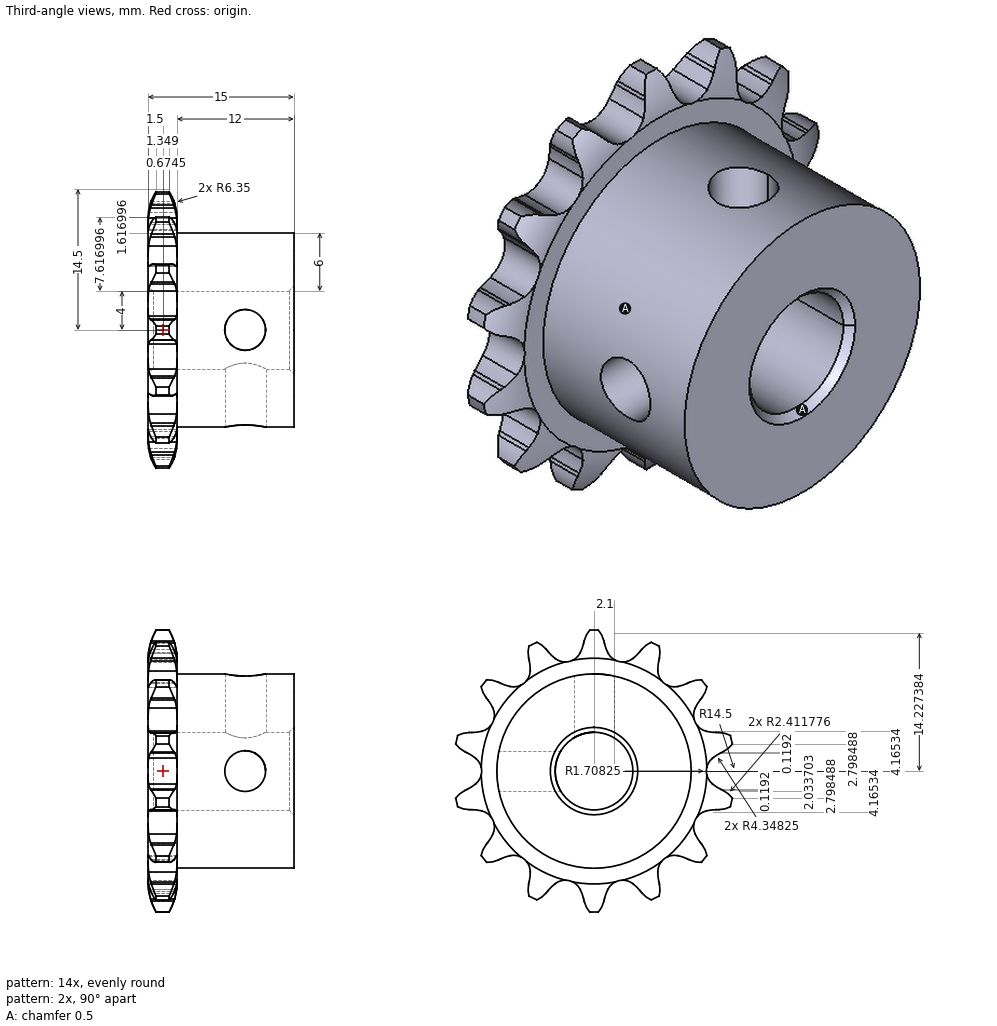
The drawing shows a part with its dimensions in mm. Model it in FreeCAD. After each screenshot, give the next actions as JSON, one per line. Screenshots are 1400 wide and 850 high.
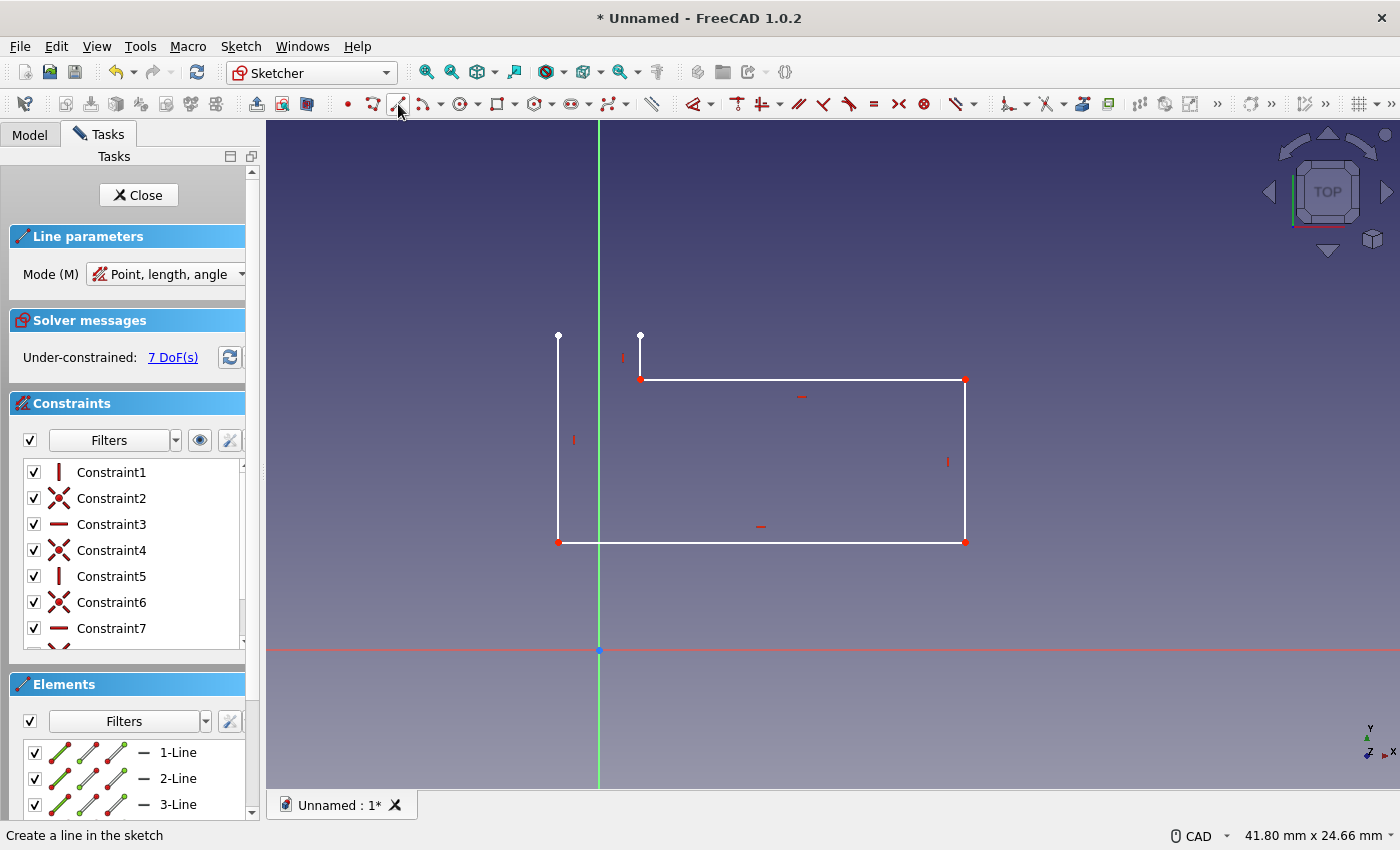
{"action": "left_click", "coordinate": [617, 257]}
{"action": "left_click", "coordinate": [581, 257]}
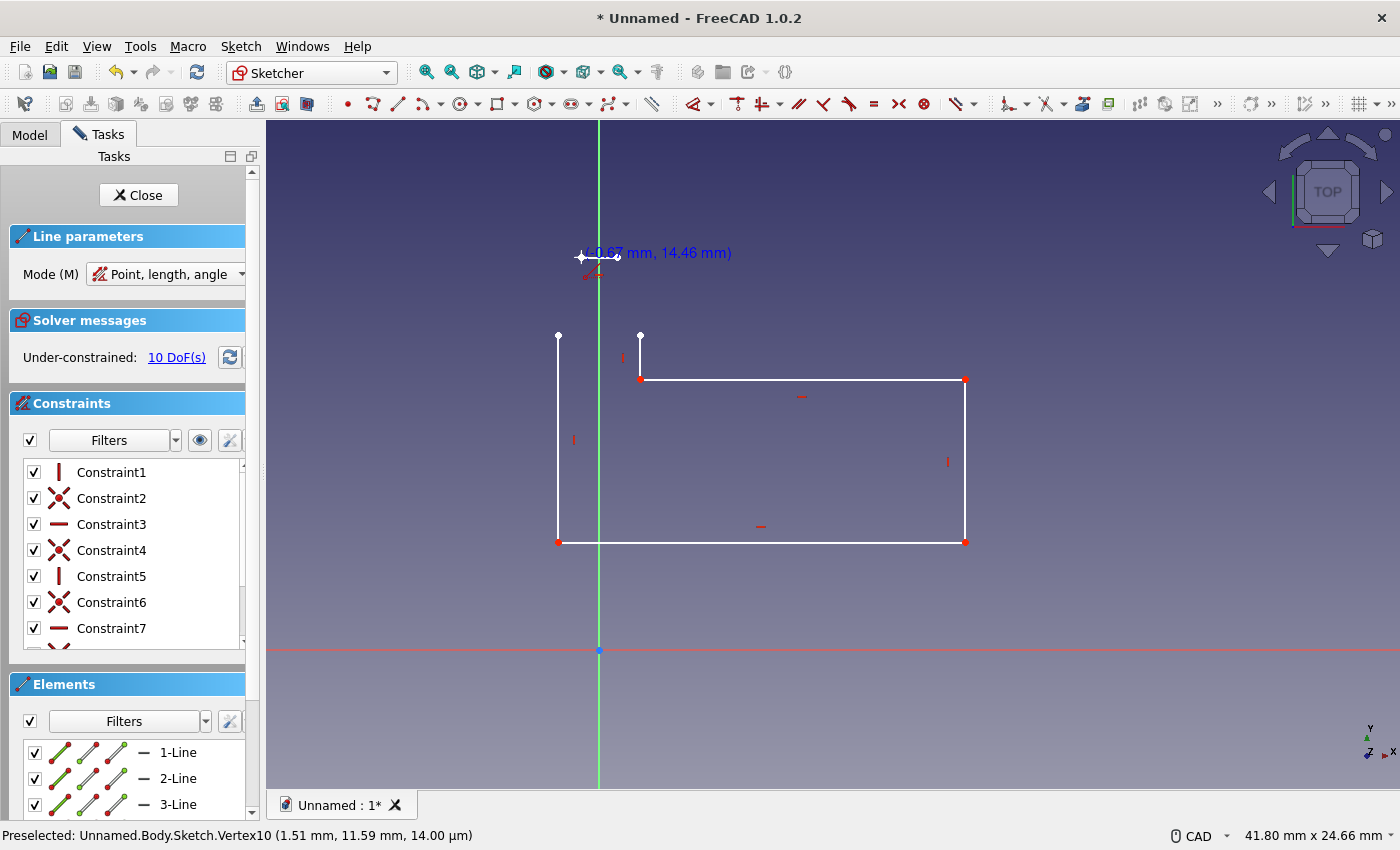
{"action": "key", "text": "g 3 a"}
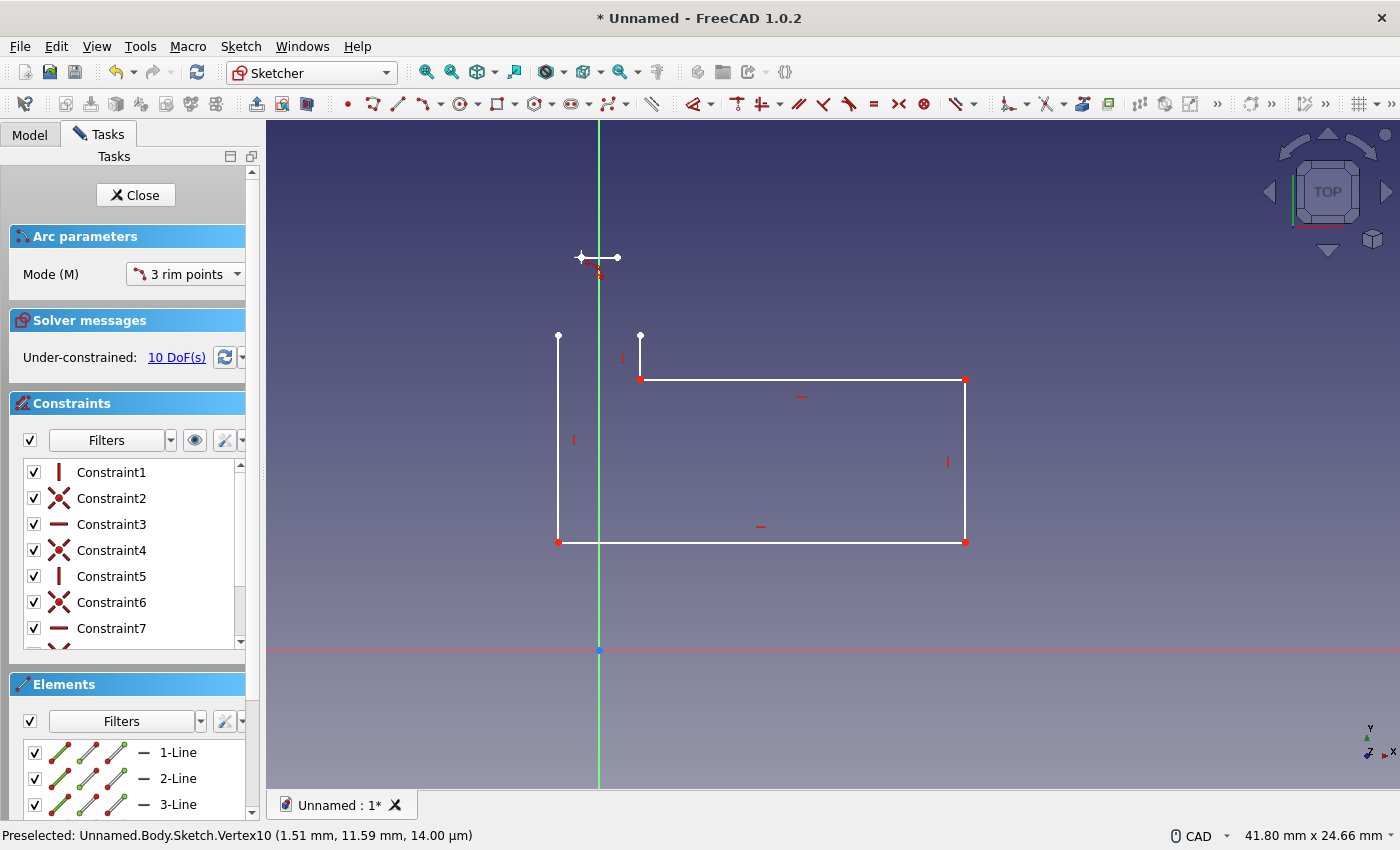
{"action": "left_click", "coordinate": [640, 336]}
{"action": "left_click", "coordinate": [617, 258]}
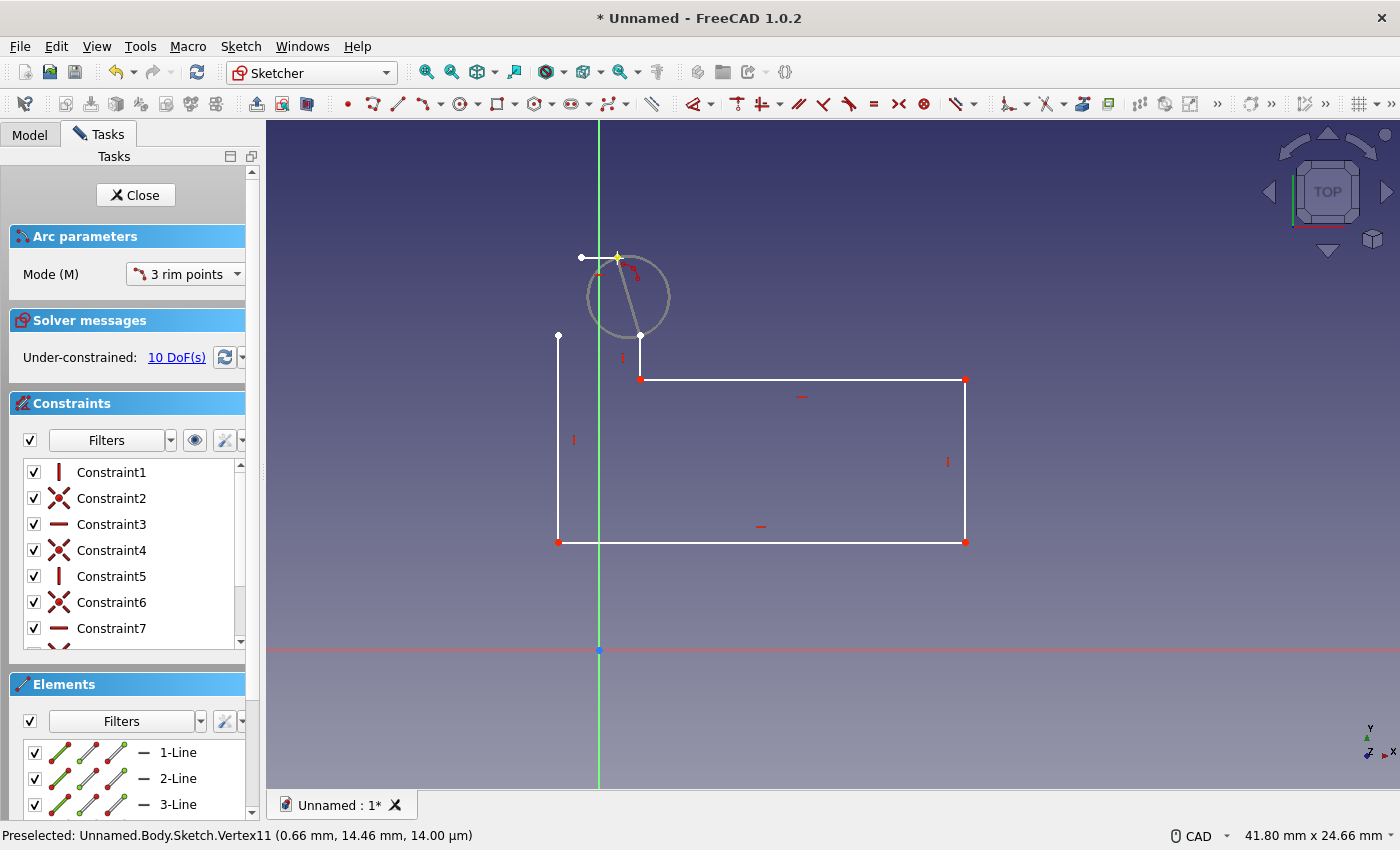
{"action": "scroll", "coordinate": [633, 295], "scroll_direction": "up", "scroll_amount": 6}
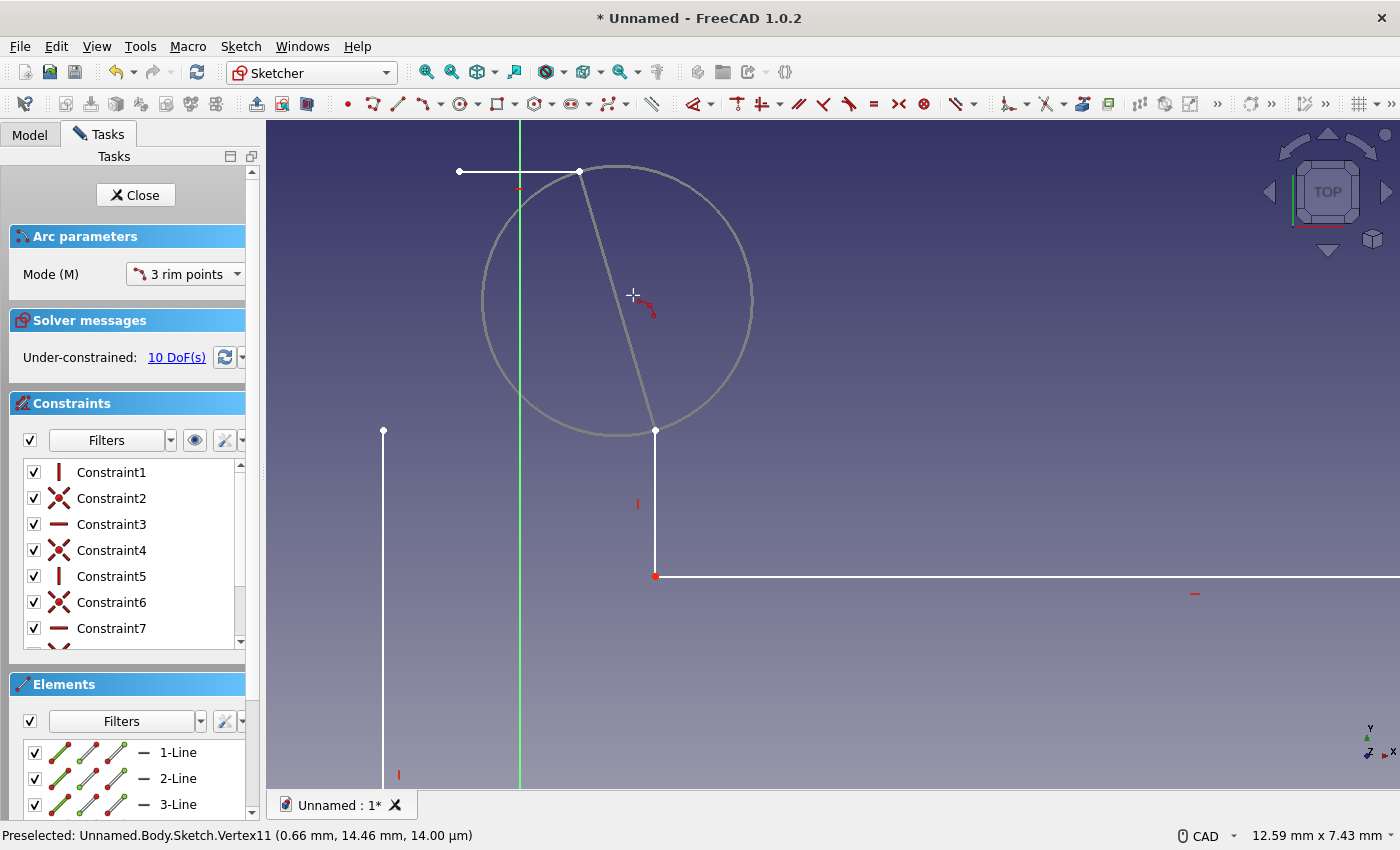
{"action": "left_click", "coordinate": [633, 293]}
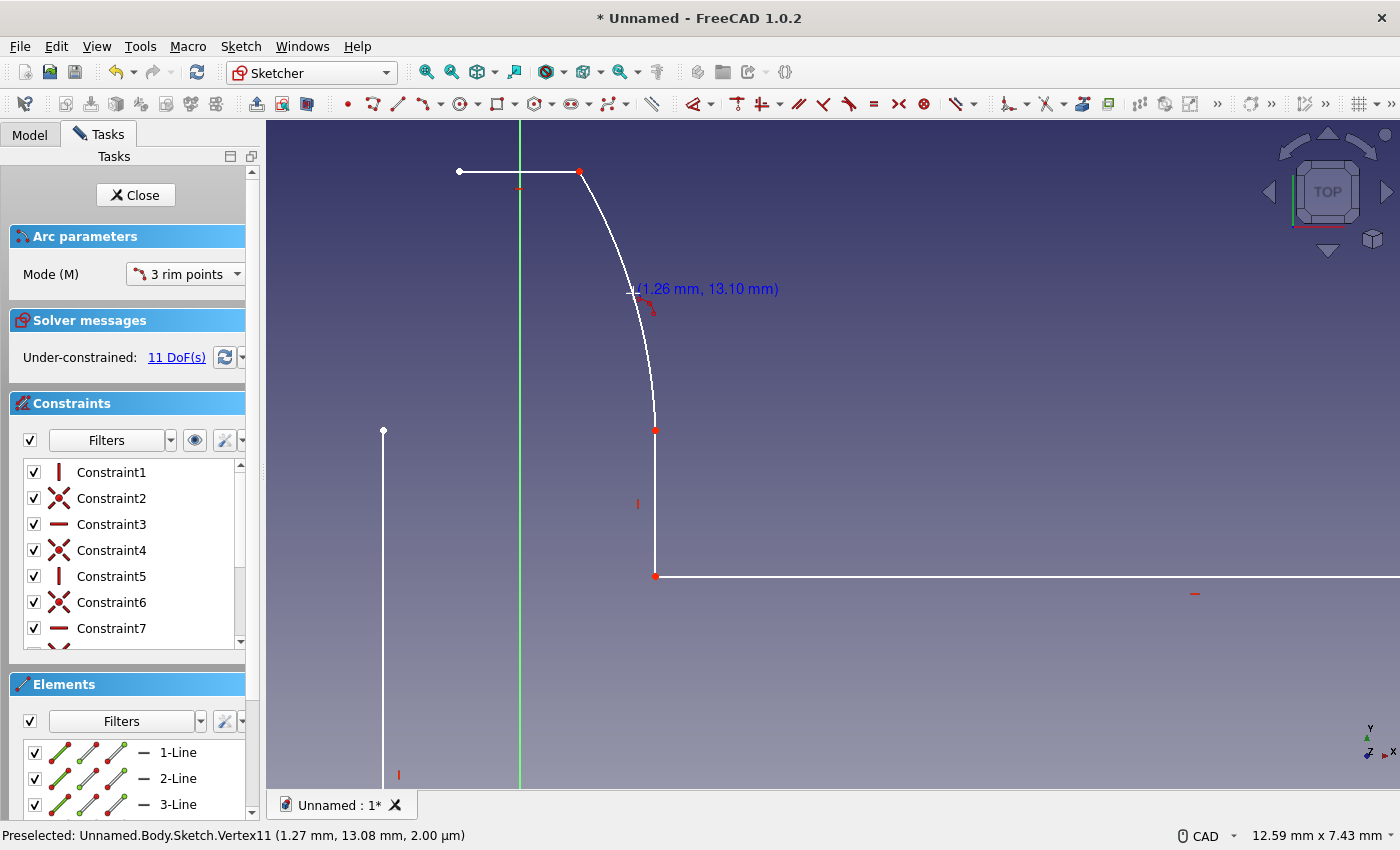
{"action": "left_click", "coordinate": [460, 172]}
{"action": "left_click", "coordinate": [383, 431]}
{"action": "left_click", "coordinate": [406, 293]}
{"action": "key", "text": "Escape"}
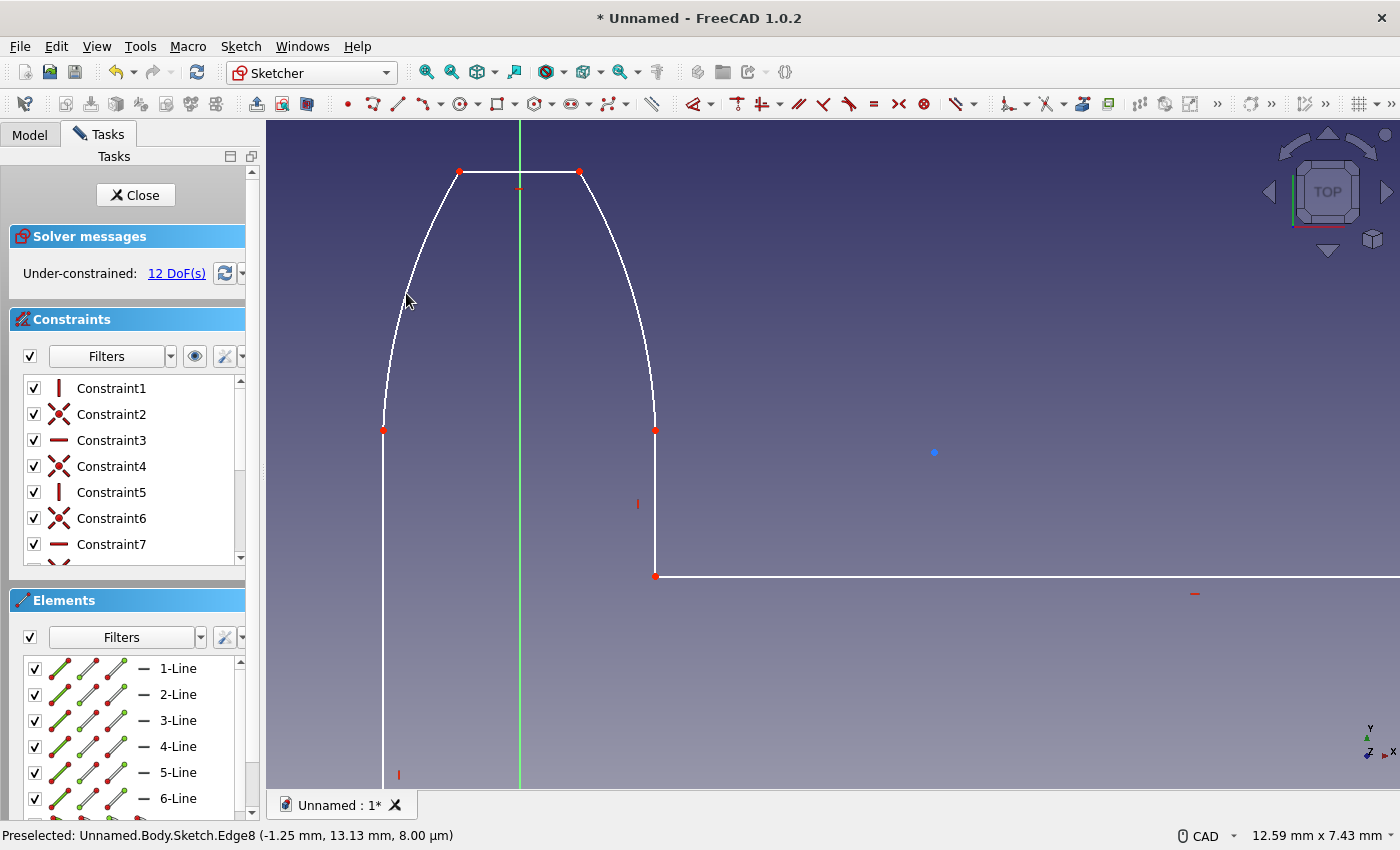
{"action": "left_click", "coordinate": [646, 349]}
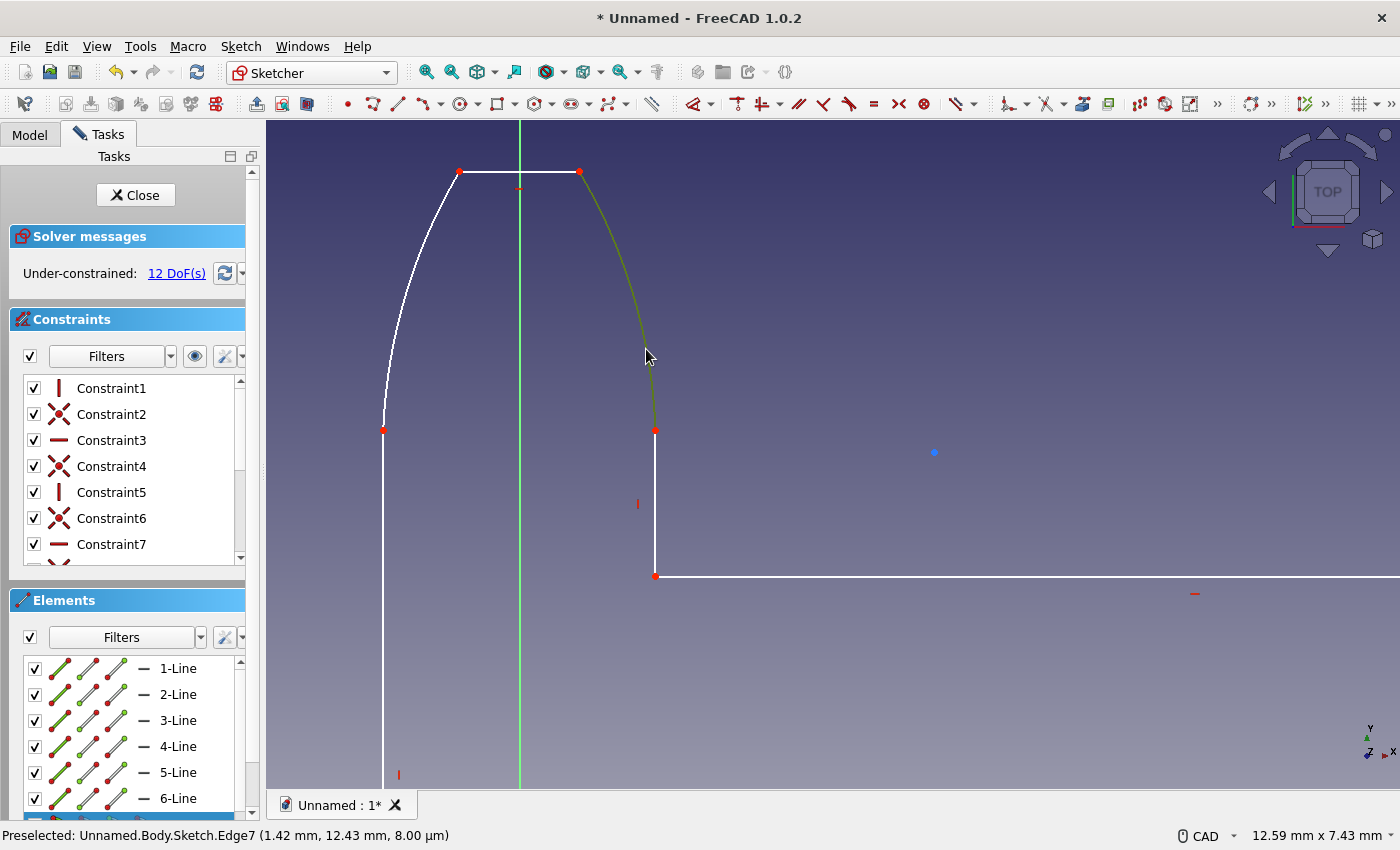
{"action": "left_click", "coordinate": [423, 245]}